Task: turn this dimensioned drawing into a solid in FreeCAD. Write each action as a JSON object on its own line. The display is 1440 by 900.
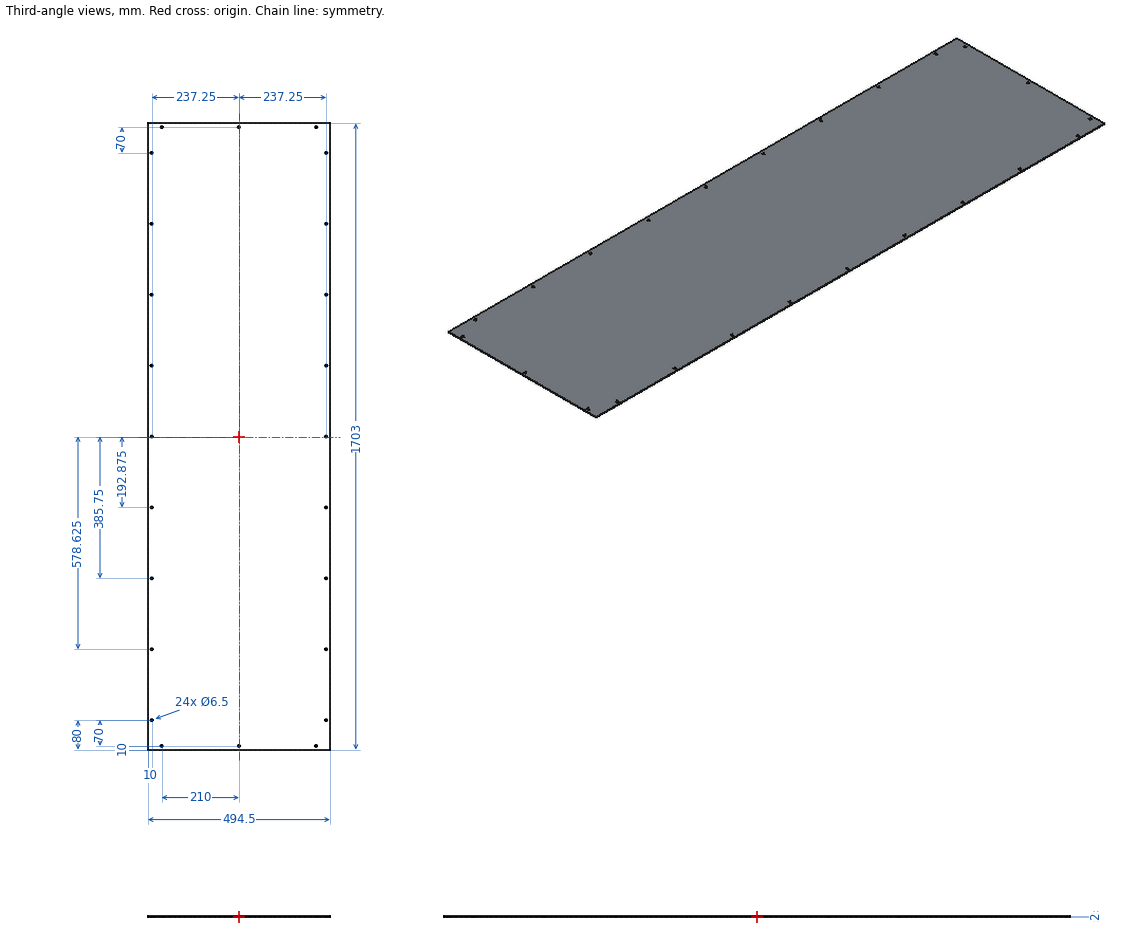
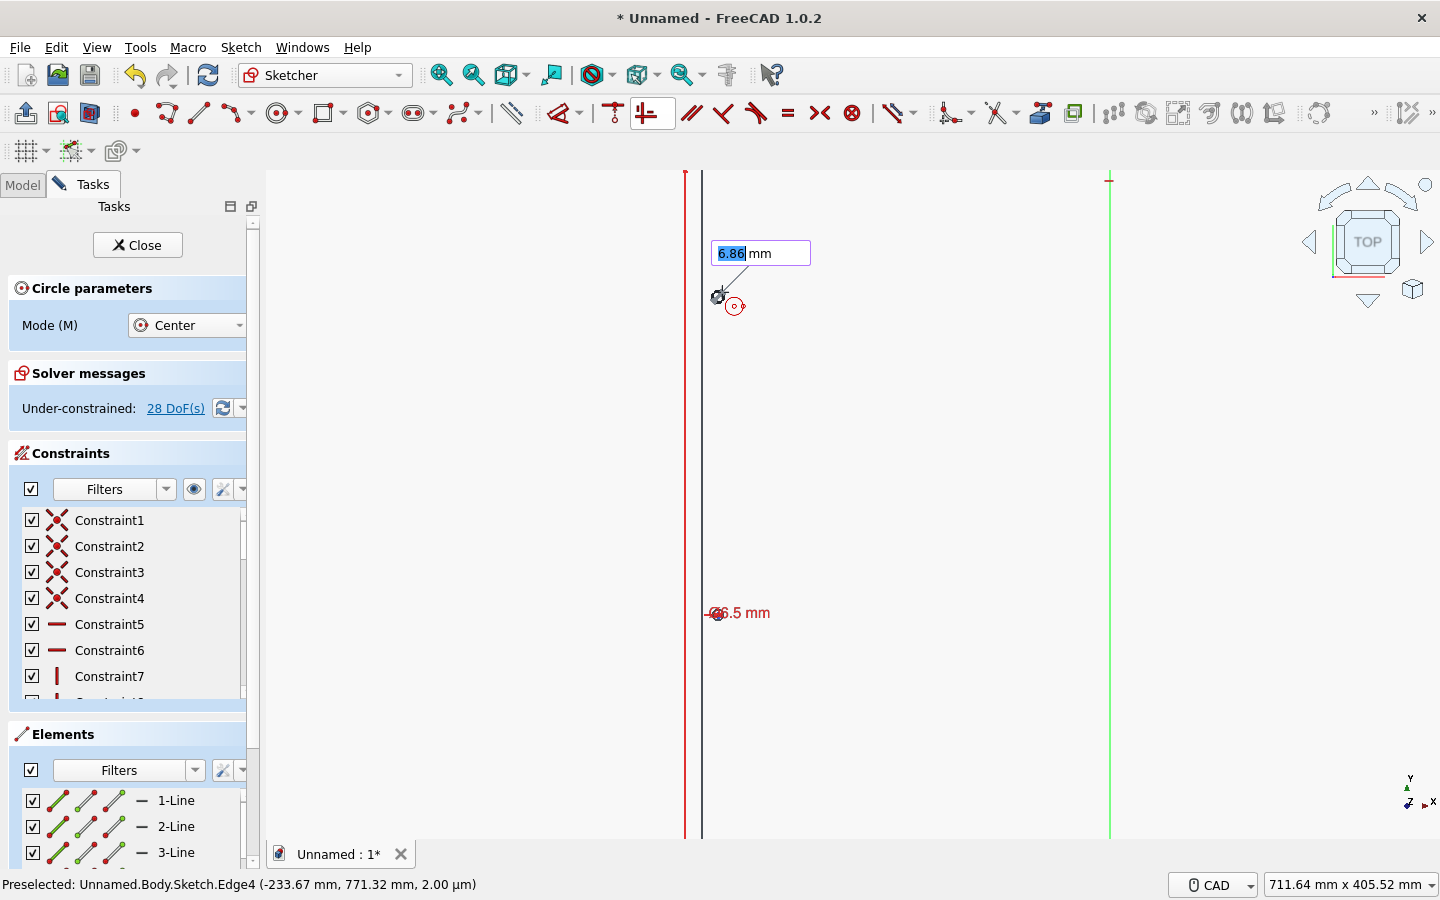
{"action": "type", "text": "6.5"}
{"action": "key", "text": "Return"}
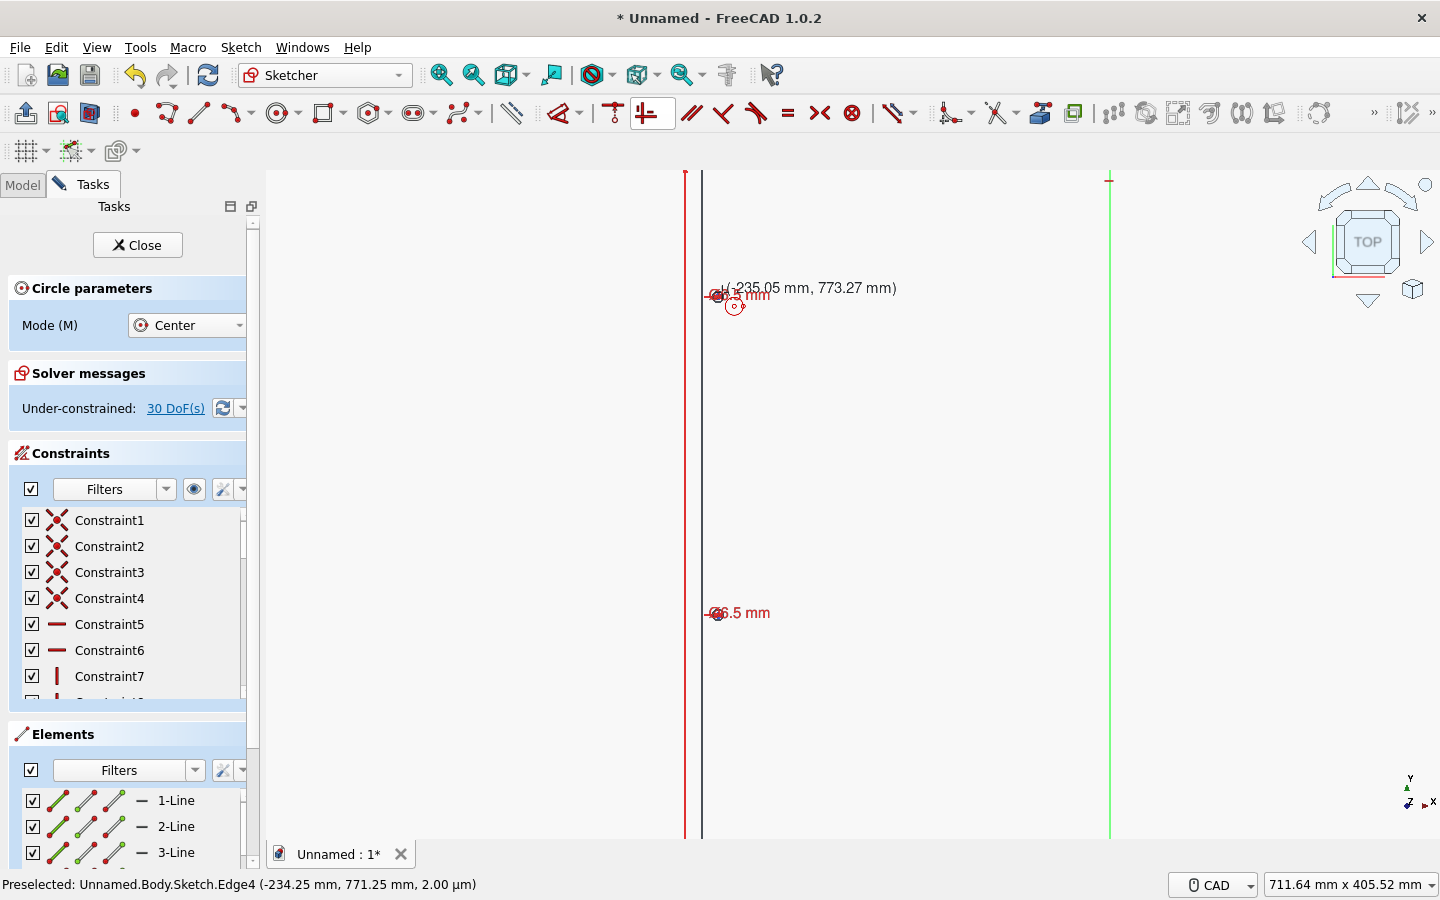
{"action": "scroll", "coordinate": [720, 294], "scroll_direction": "down", "scroll_amount": 9}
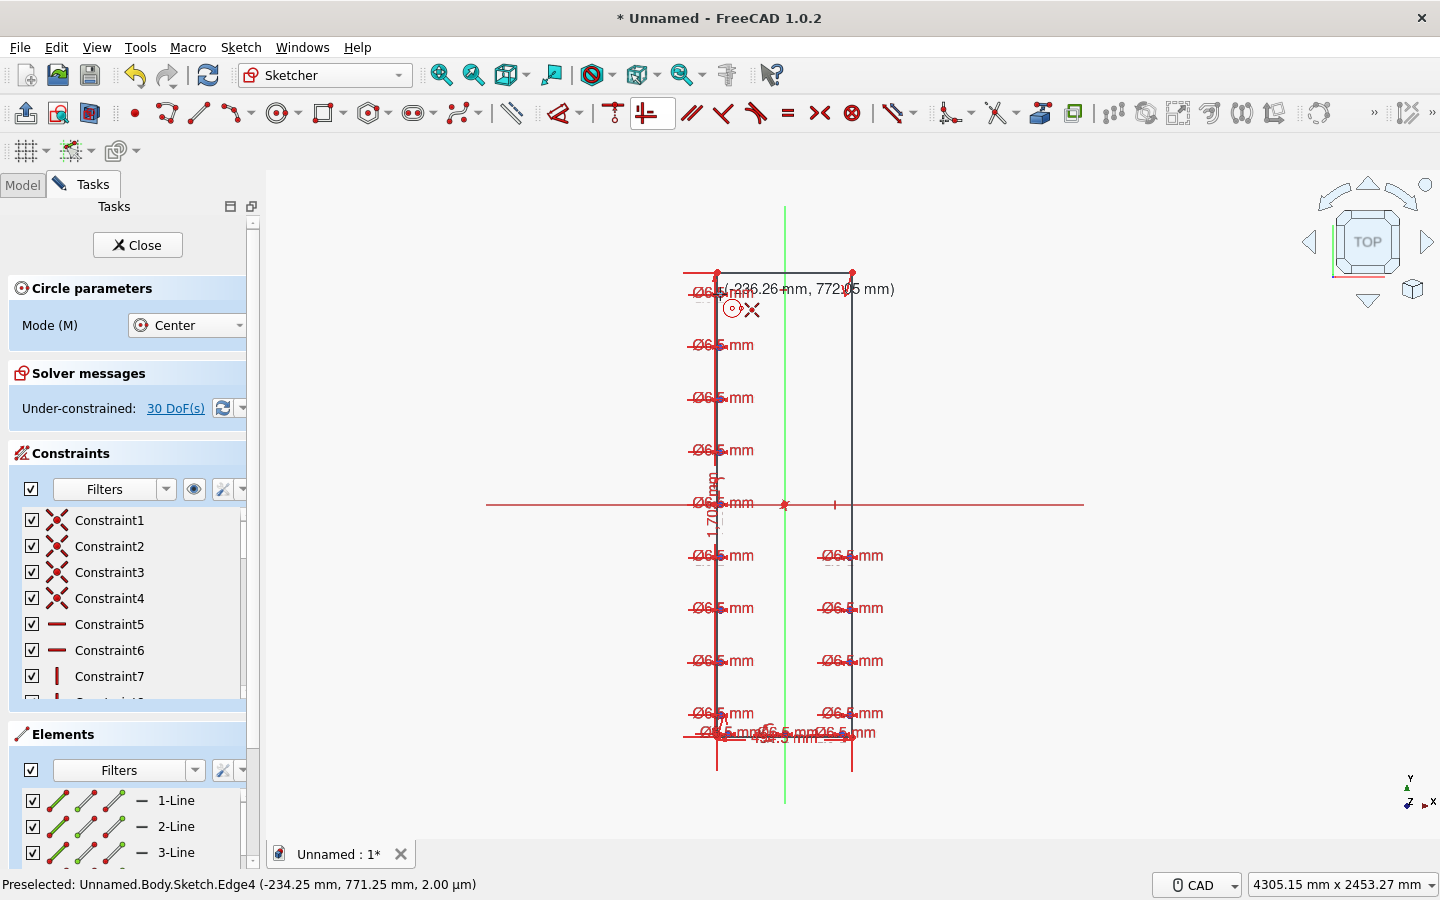
{"action": "scroll", "coordinate": [727, 275], "scroll_direction": "up", "scroll_amount": 17}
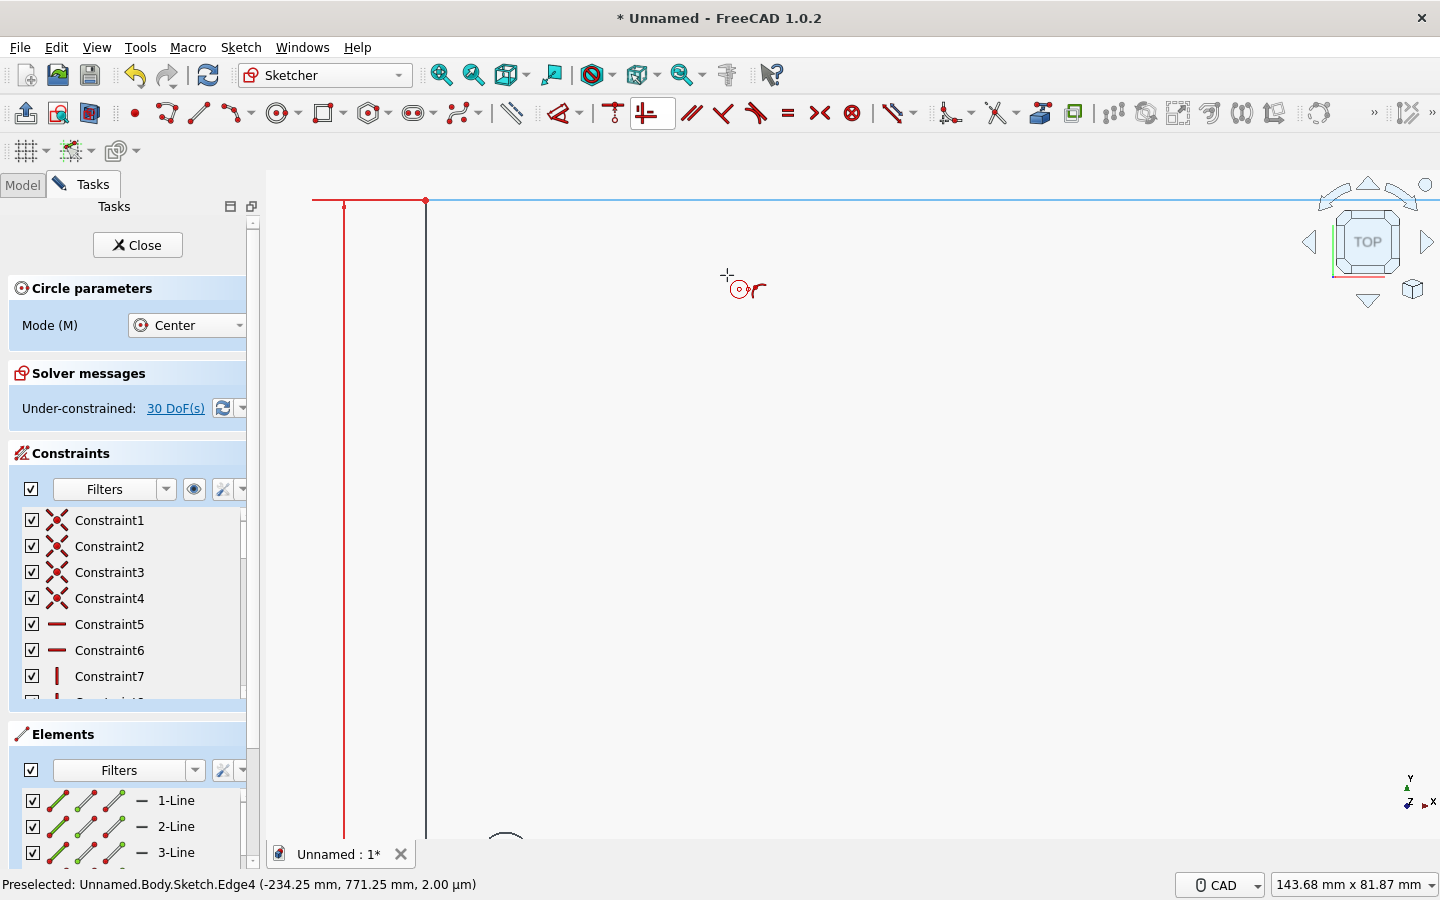
{"action": "scroll", "coordinate": [727, 275], "scroll_direction": "down", "scroll_amount": 17}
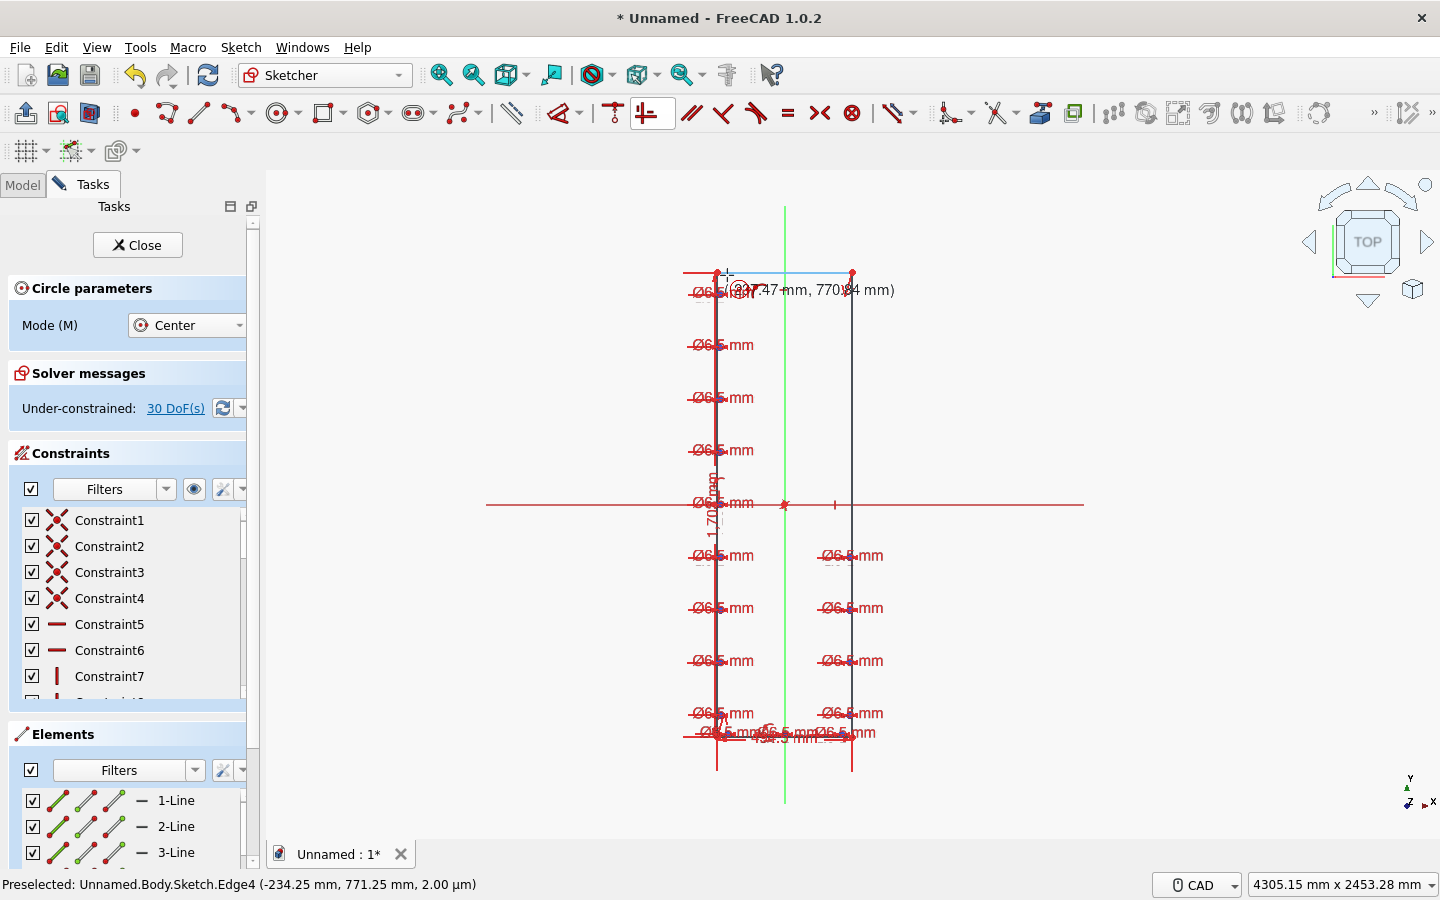
{"action": "scroll", "coordinate": [727, 275], "scroll_direction": "up", "scroll_amount": 9}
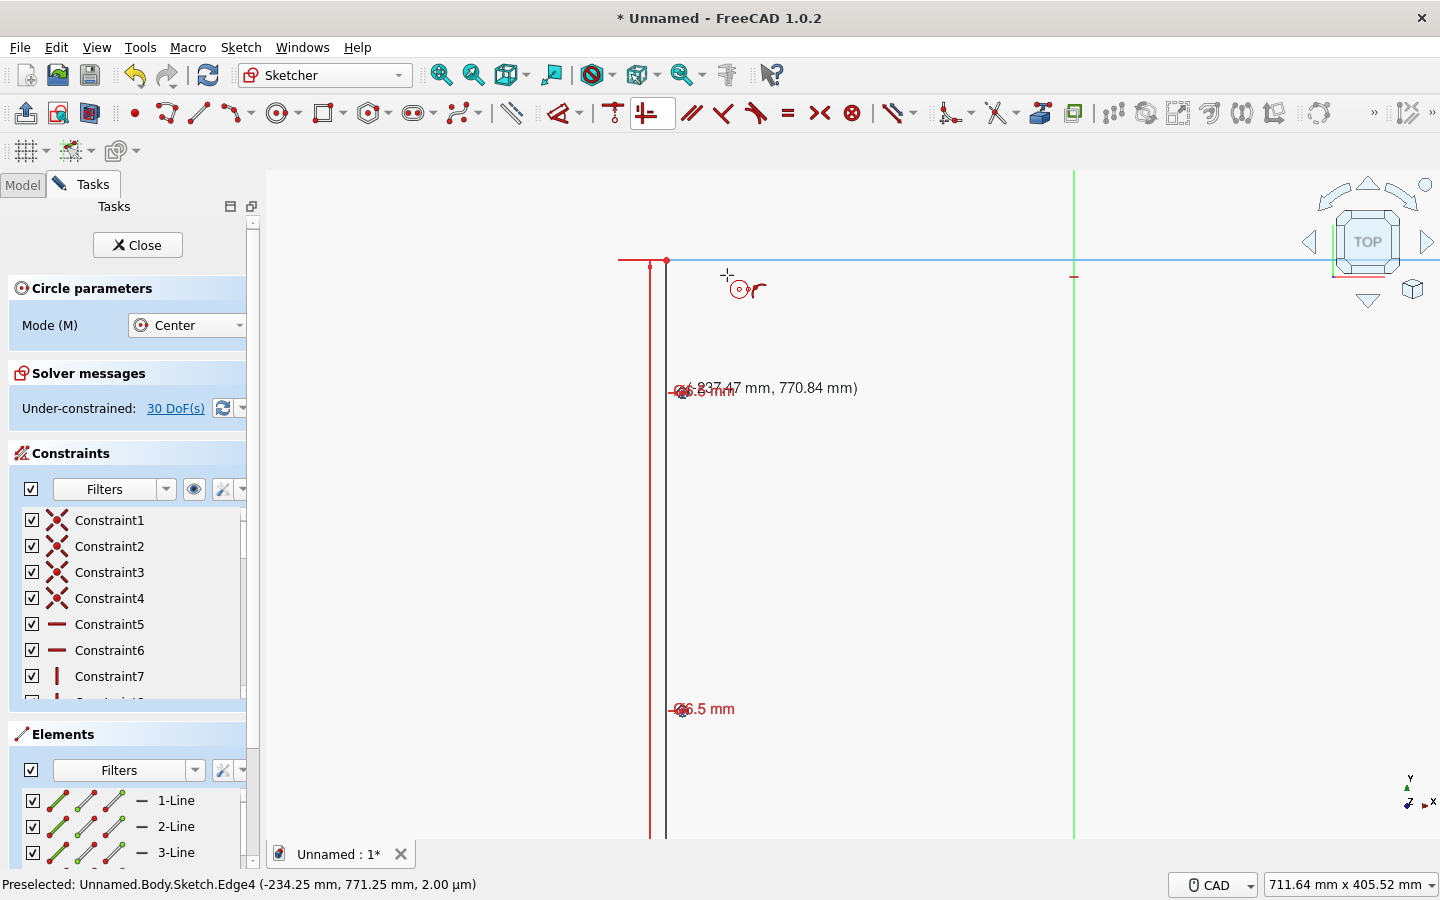
{"action": "left_click", "coordinate": [728, 277]}
{"action": "mouse_move", "coordinate": [732, 280]}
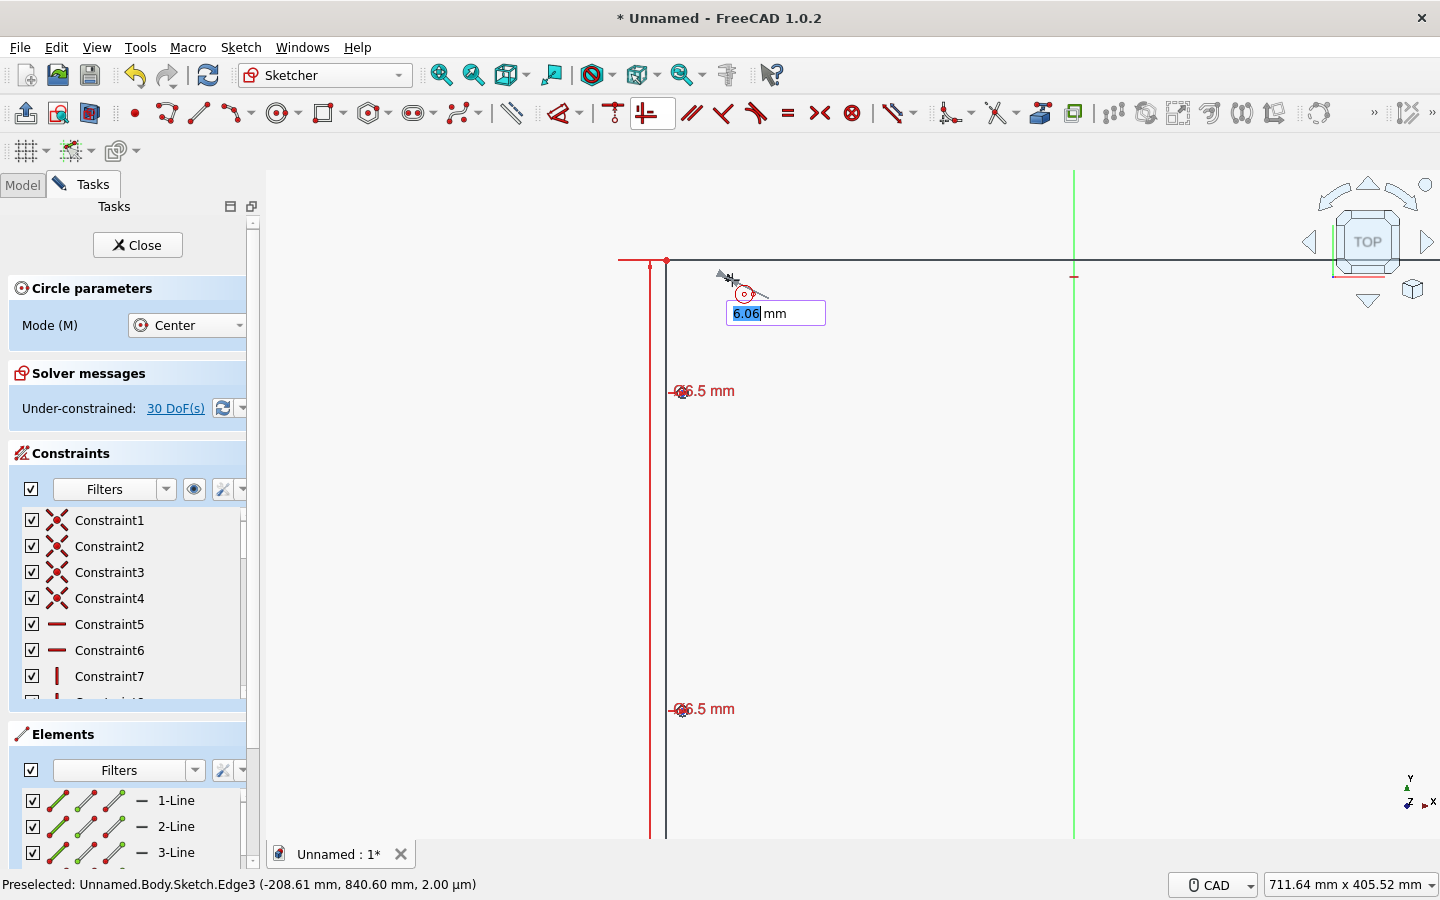
{"action": "type", "text": "6.5"}
{"action": "key", "text": "Return"}